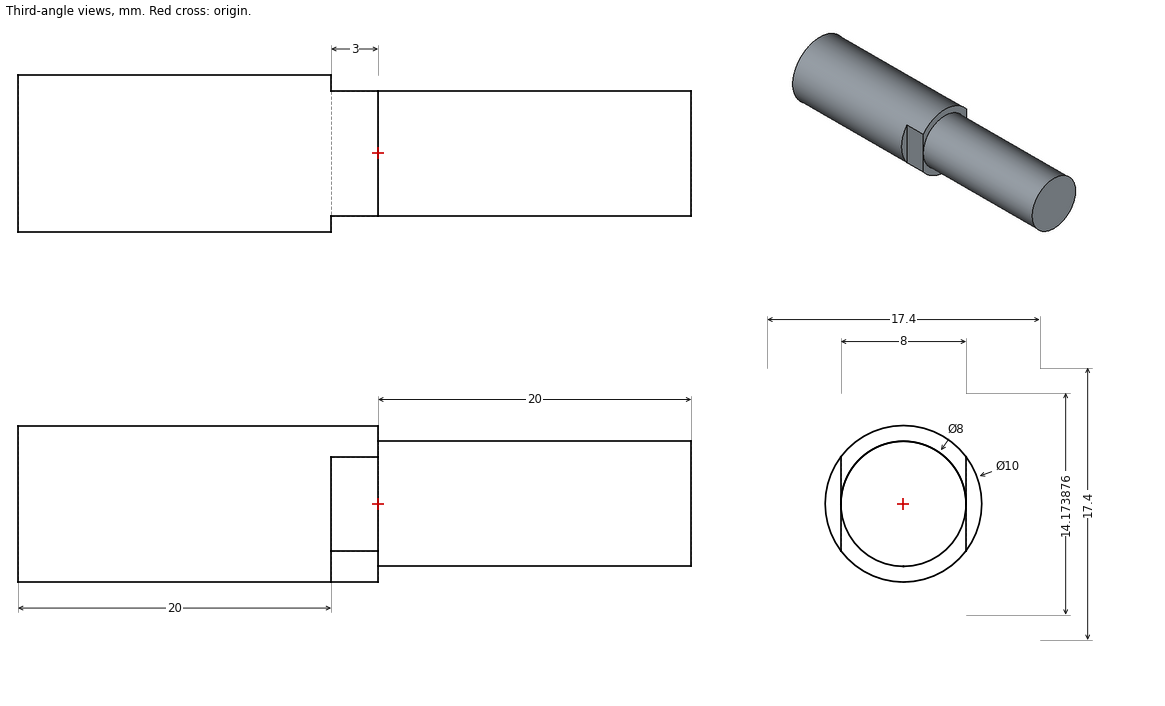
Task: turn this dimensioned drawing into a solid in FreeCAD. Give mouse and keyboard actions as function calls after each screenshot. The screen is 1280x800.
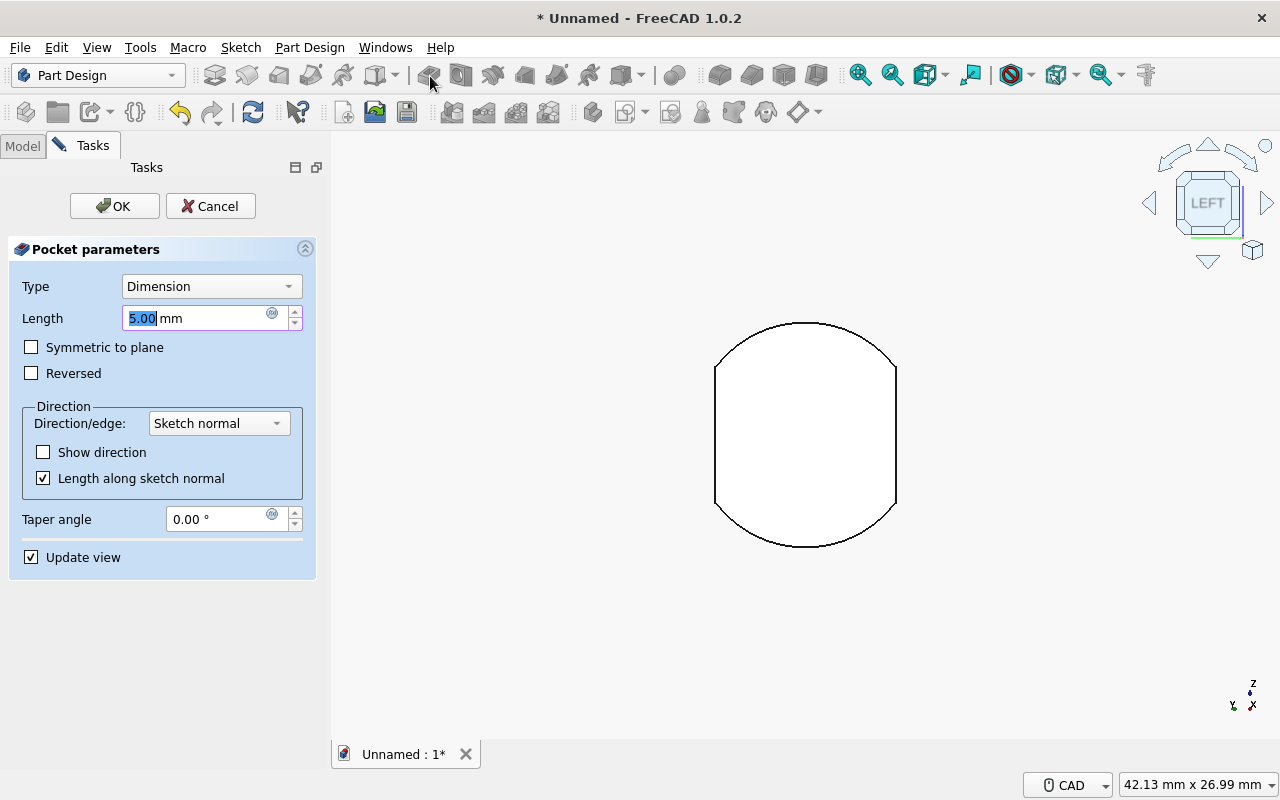
click(212, 286)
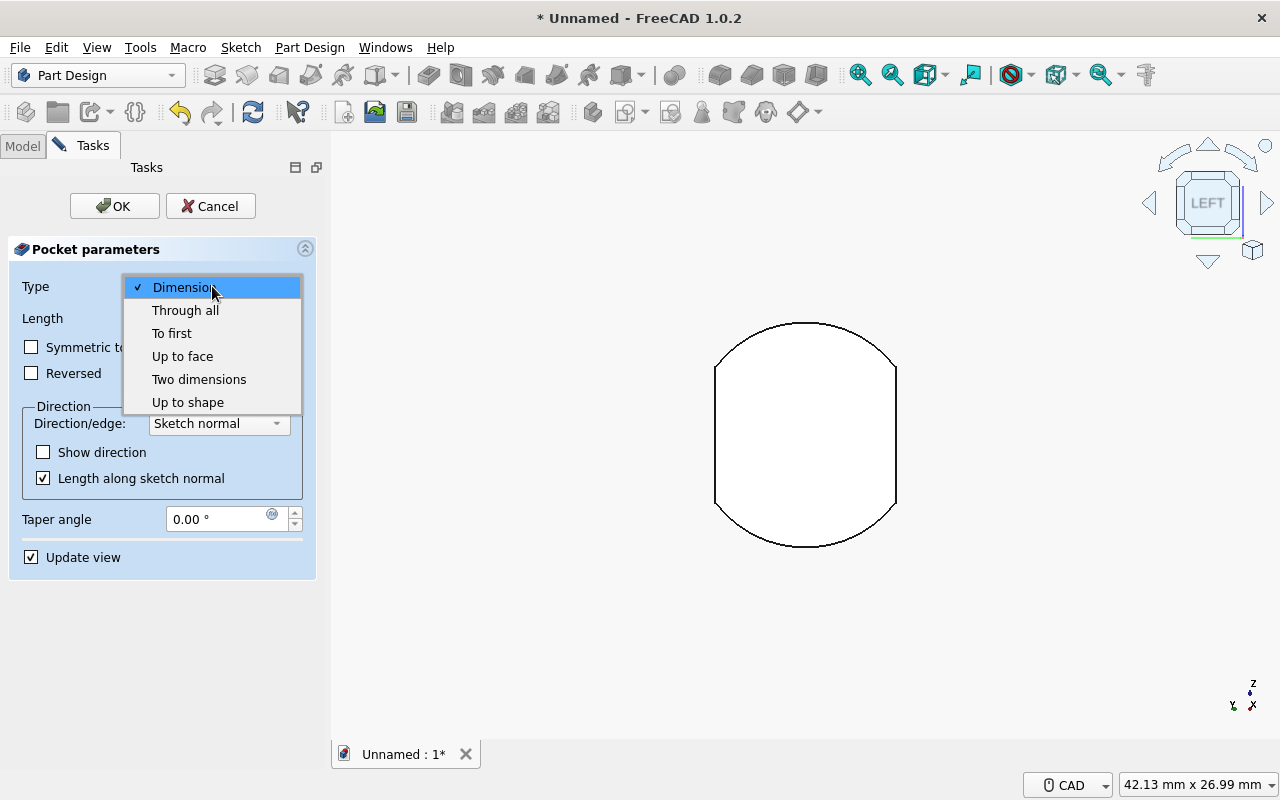
click(212, 310)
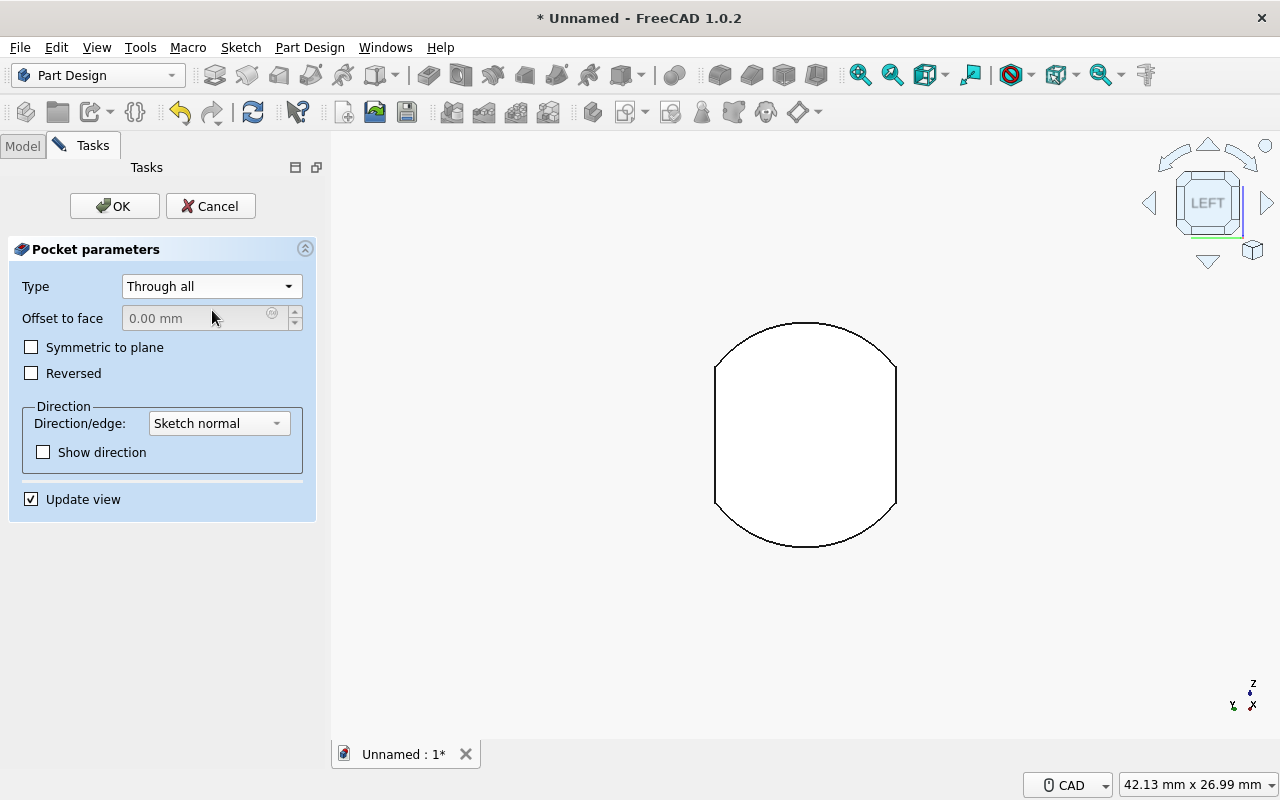
click(115, 206)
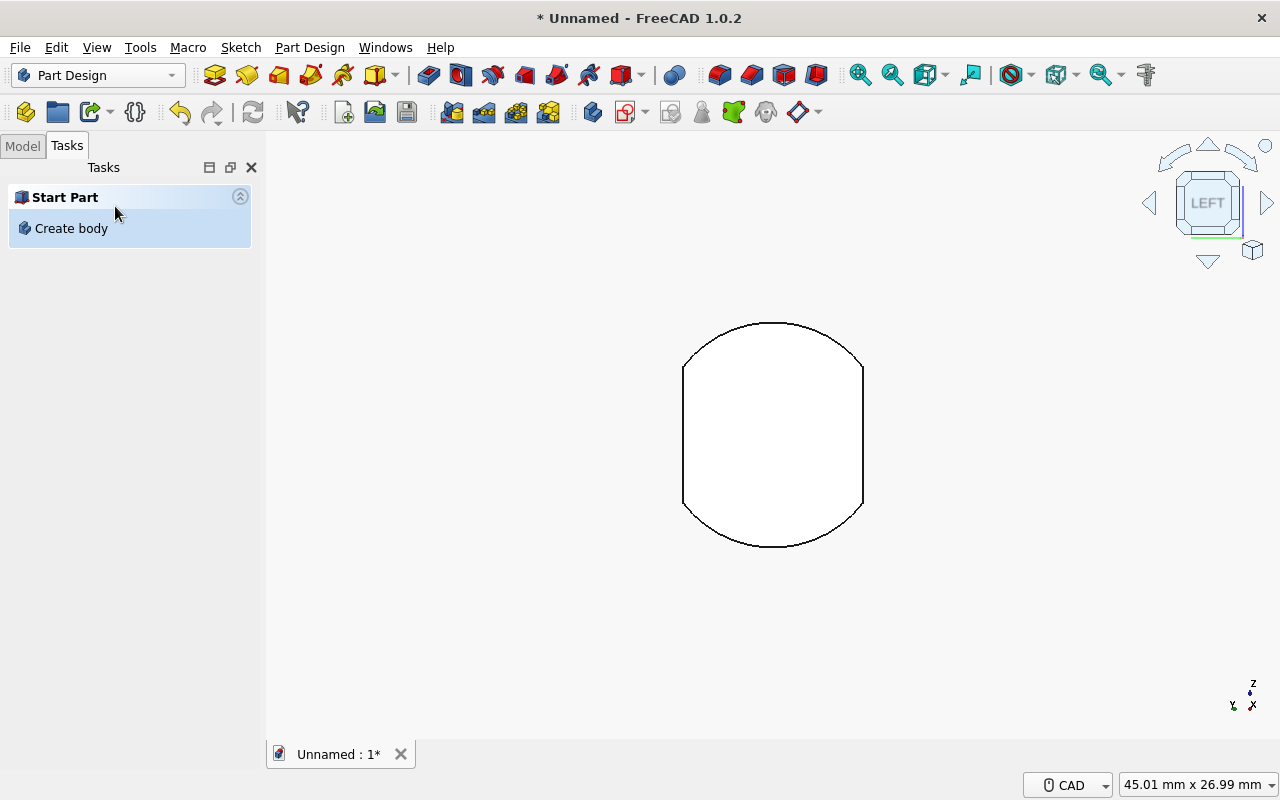
key(v)
key(f)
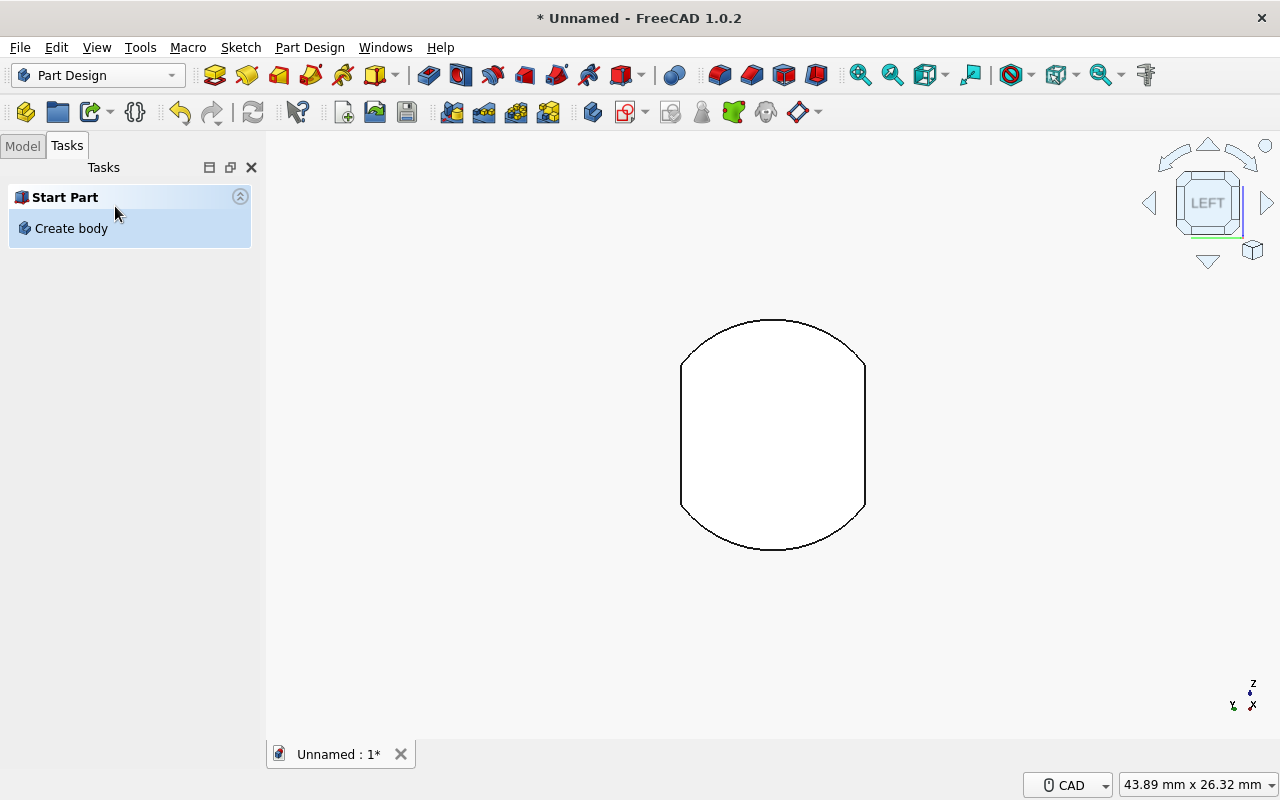
click(773, 434)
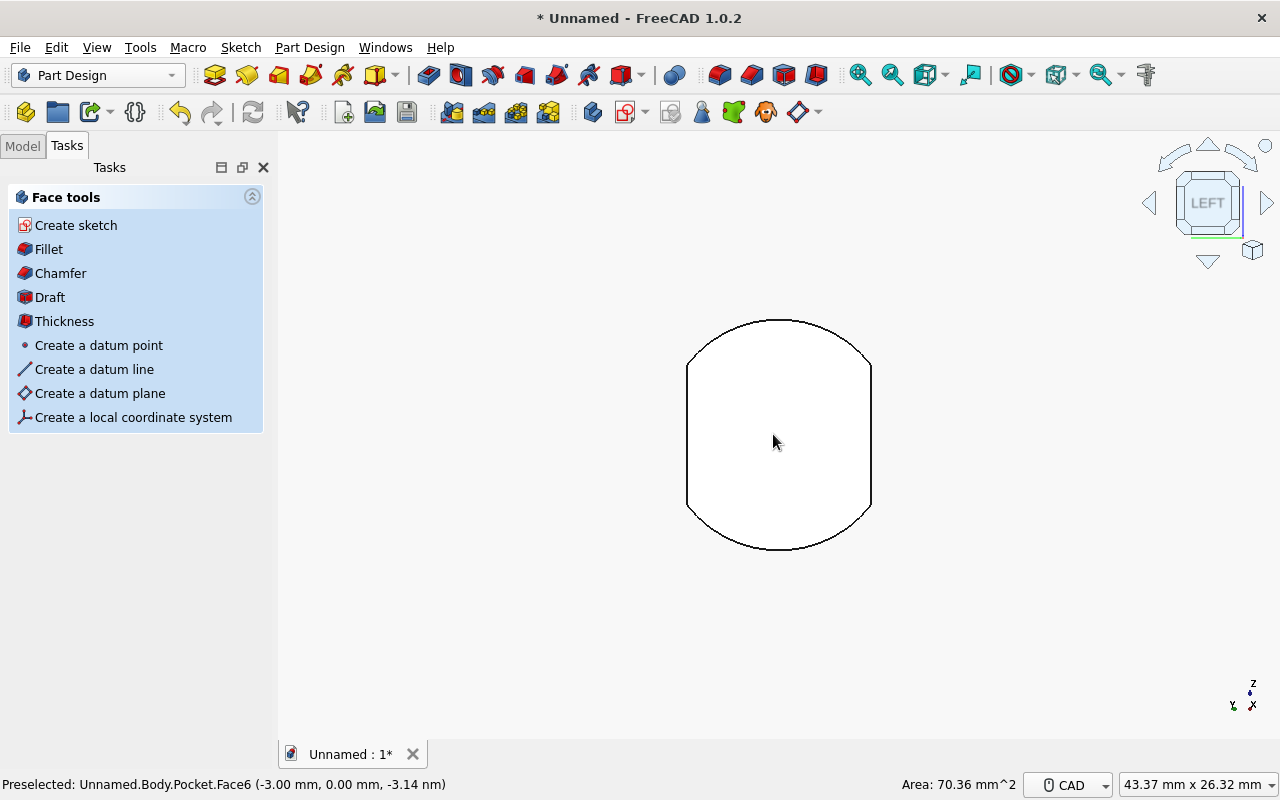
click(626, 112)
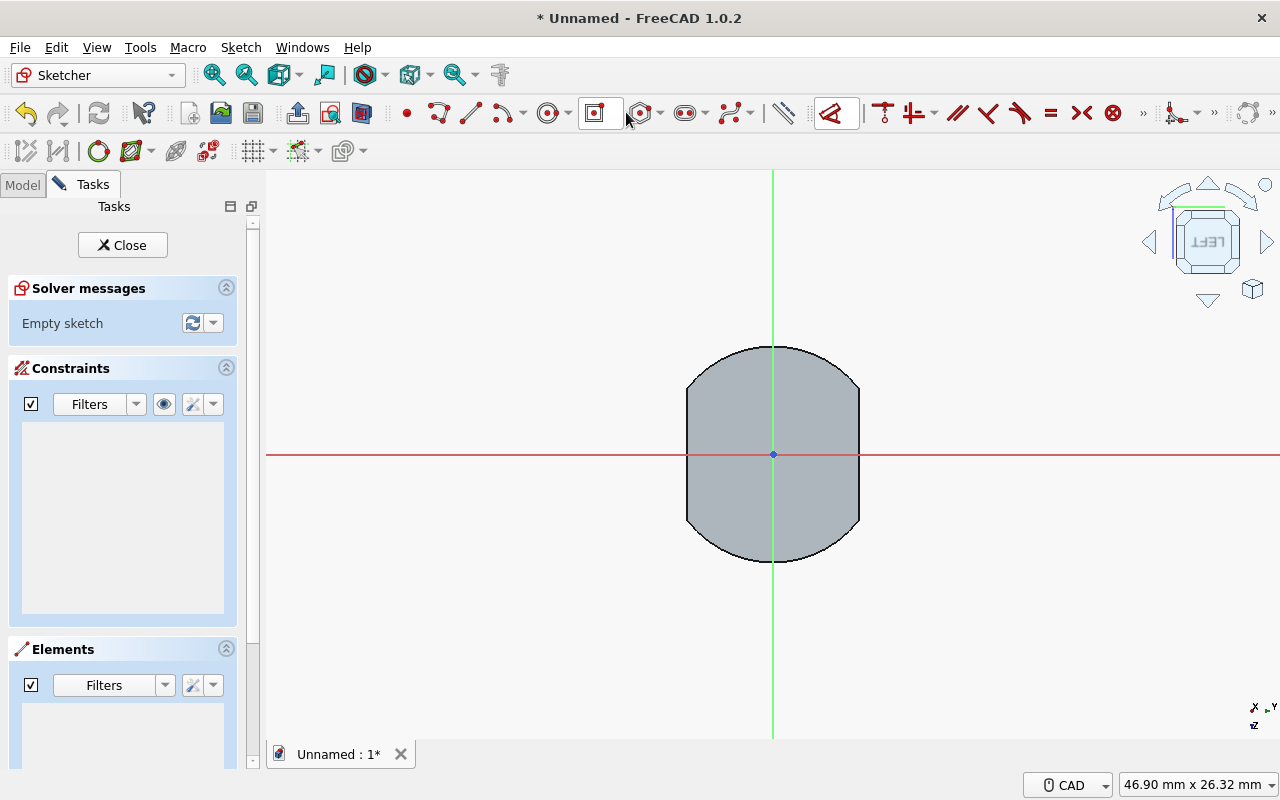
scroll(856, 454, up, 3)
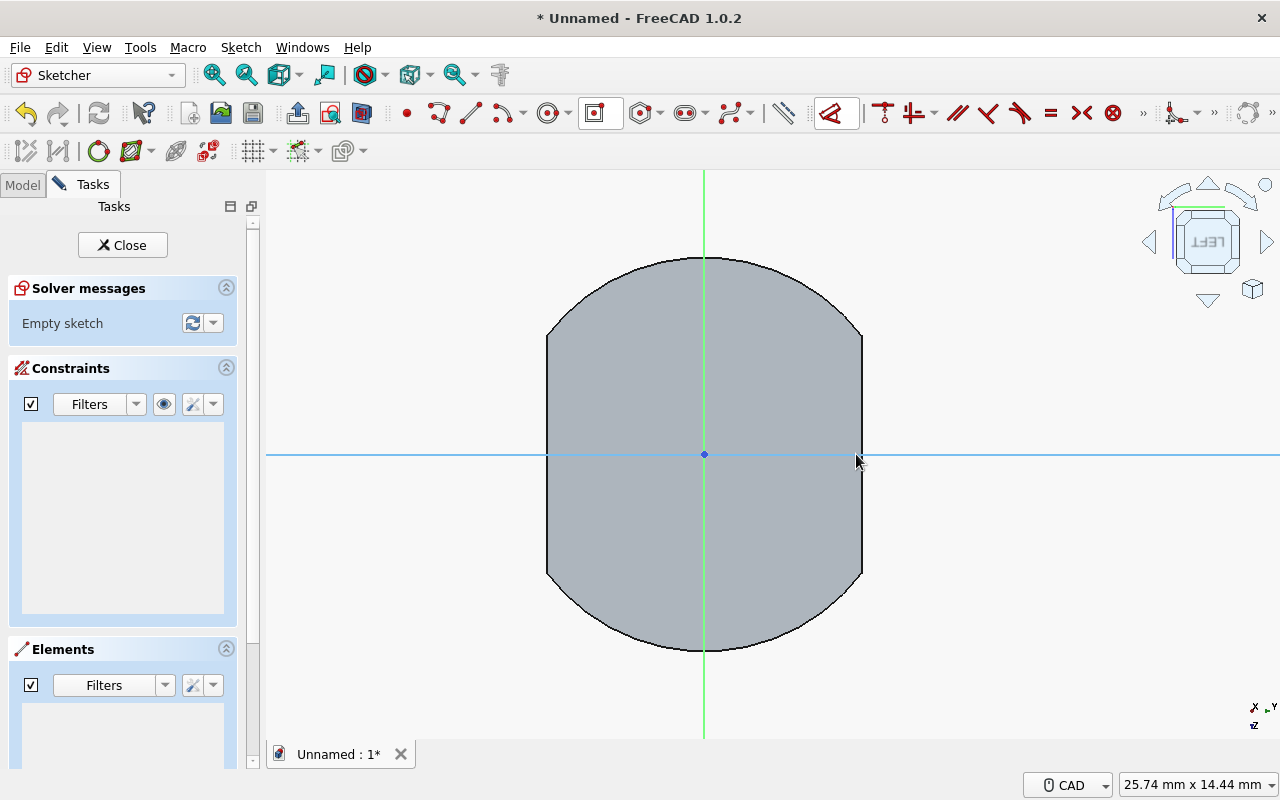
key(g)
key(c)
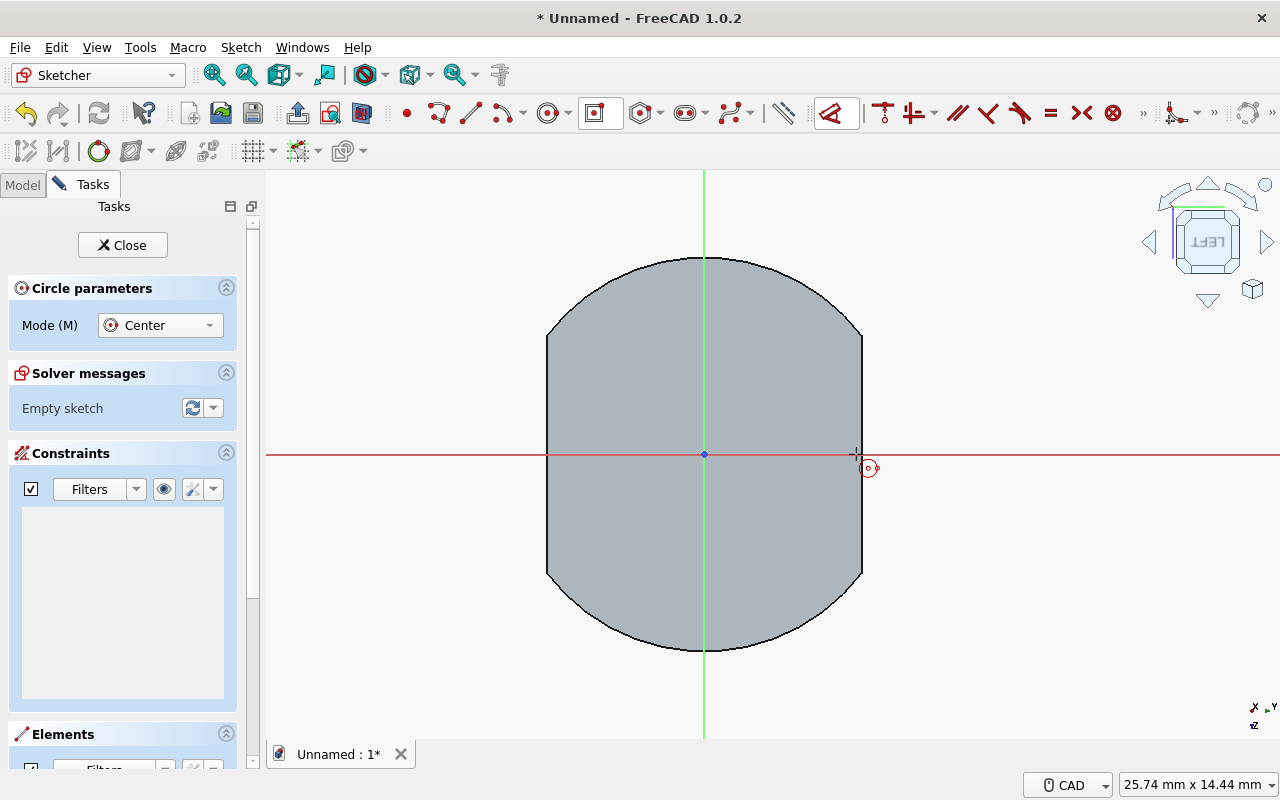
click(704, 454)
click(844, 315)
key(Escape)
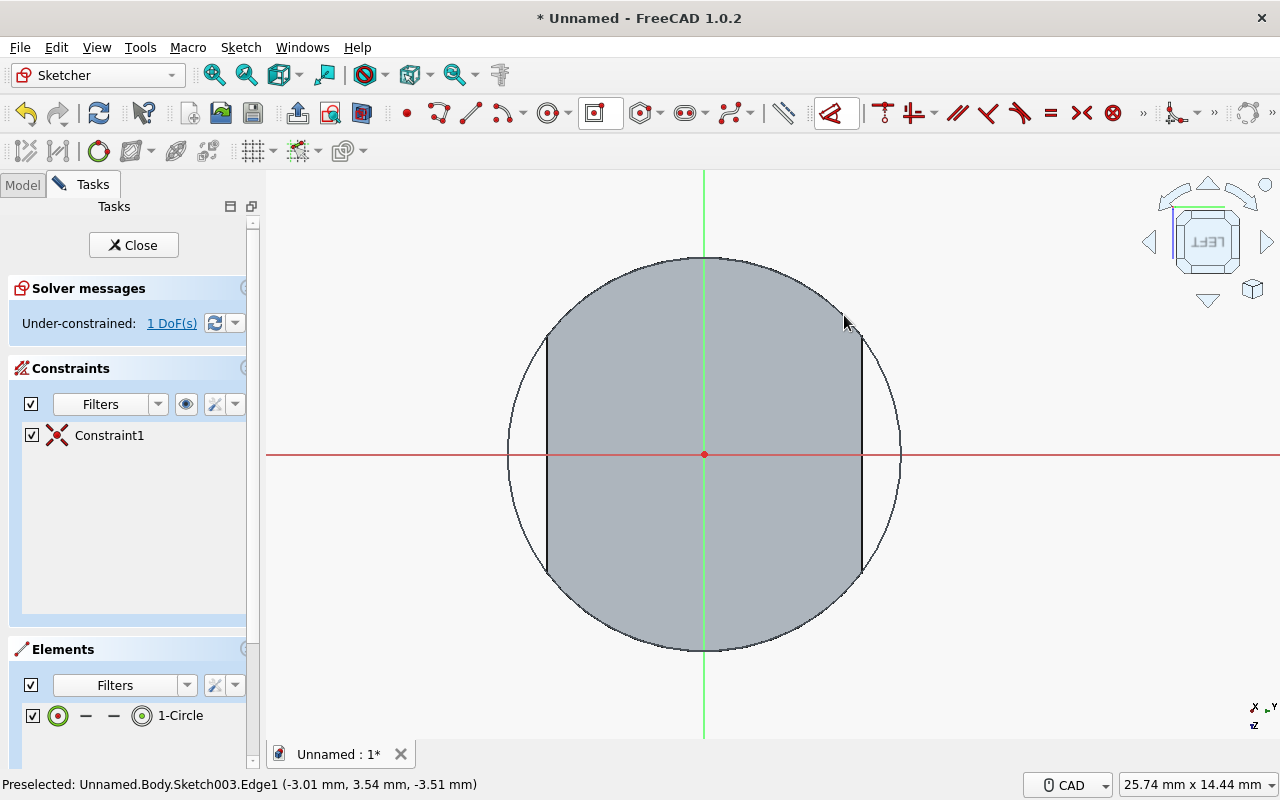
click(843, 315)